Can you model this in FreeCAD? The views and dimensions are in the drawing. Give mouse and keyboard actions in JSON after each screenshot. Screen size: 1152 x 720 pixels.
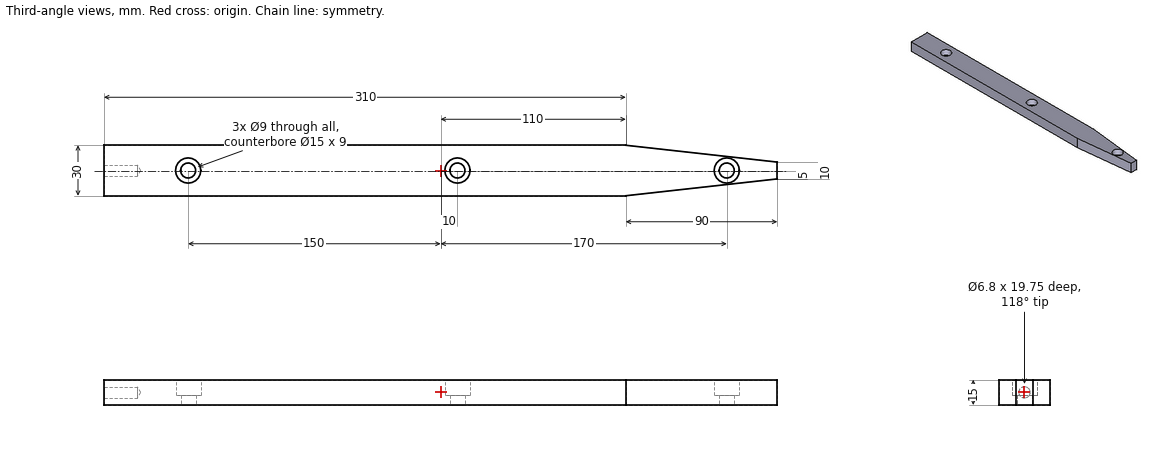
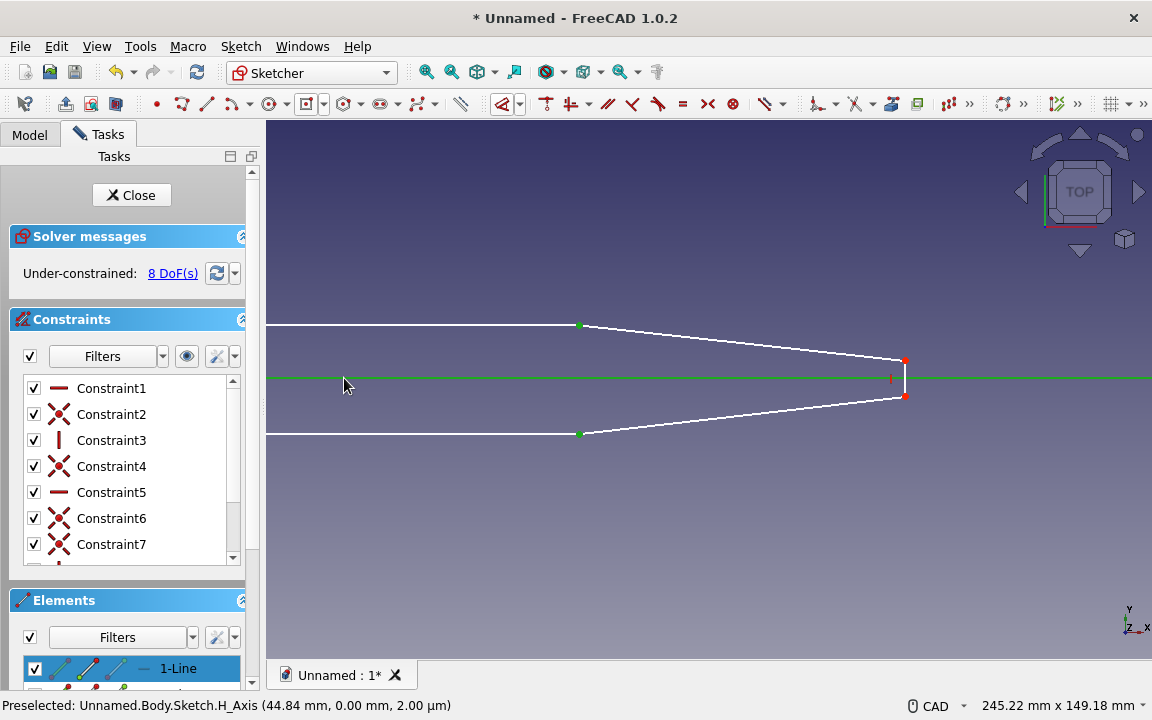
{"action": "key", "text": "s"}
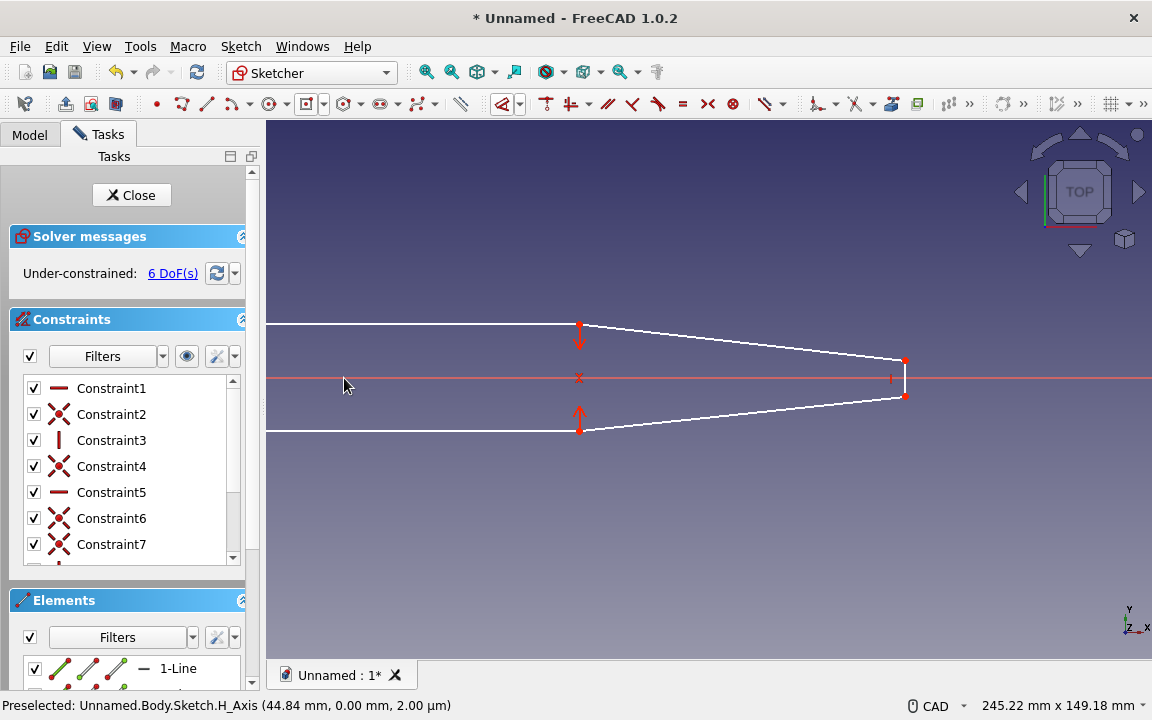
{"action": "left_click", "coordinate": [502, 104]}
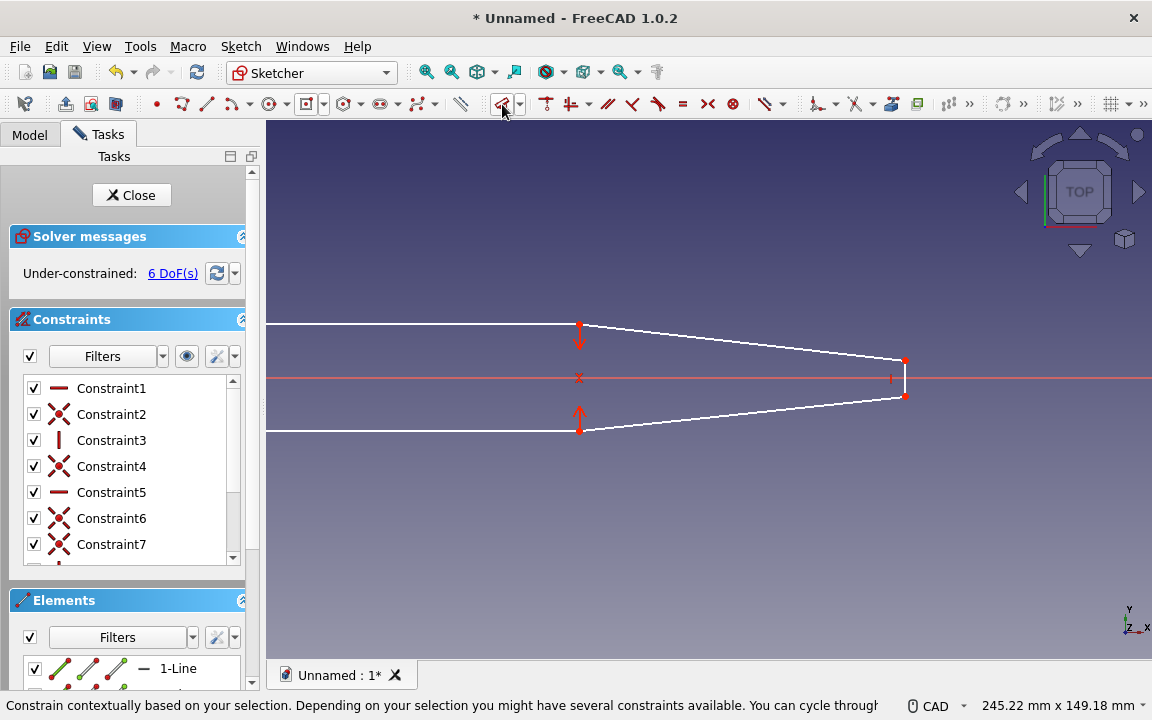
{"action": "scroll", "coordinate": [907, 396], "scroll_direction": "down", "scroll_amount": 5}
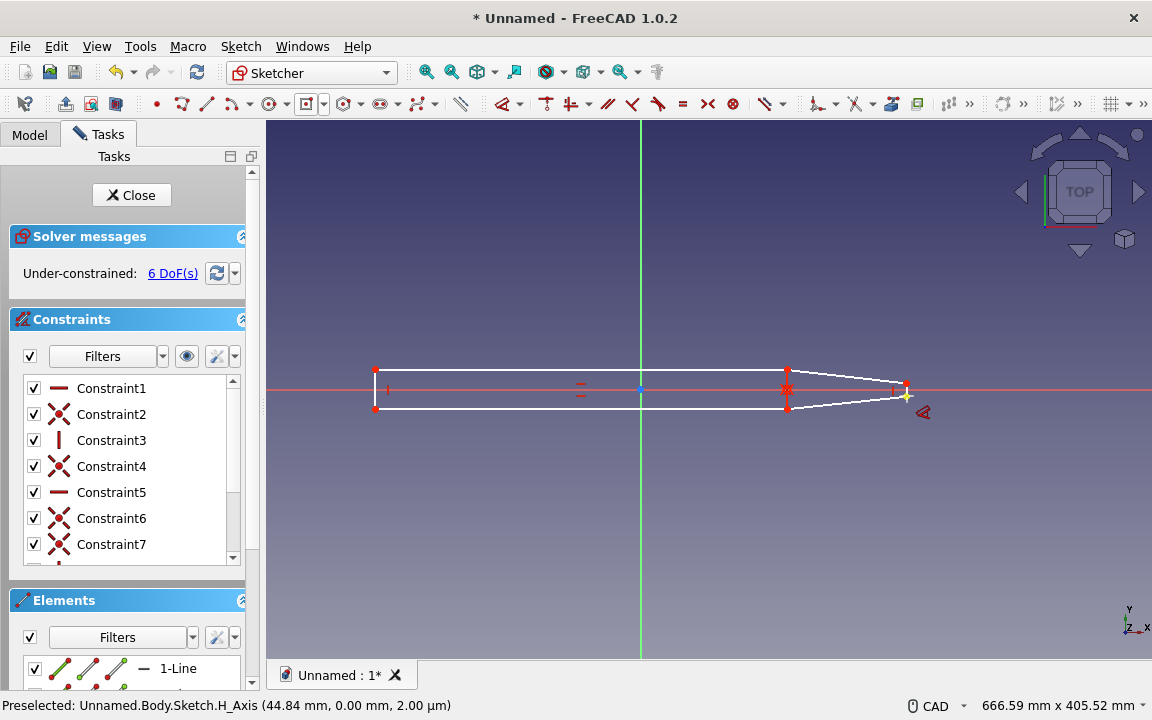
{"action": "scroll", "coordinate": [375, 382], "scroll_direction": "up", "scroll_amount": 3}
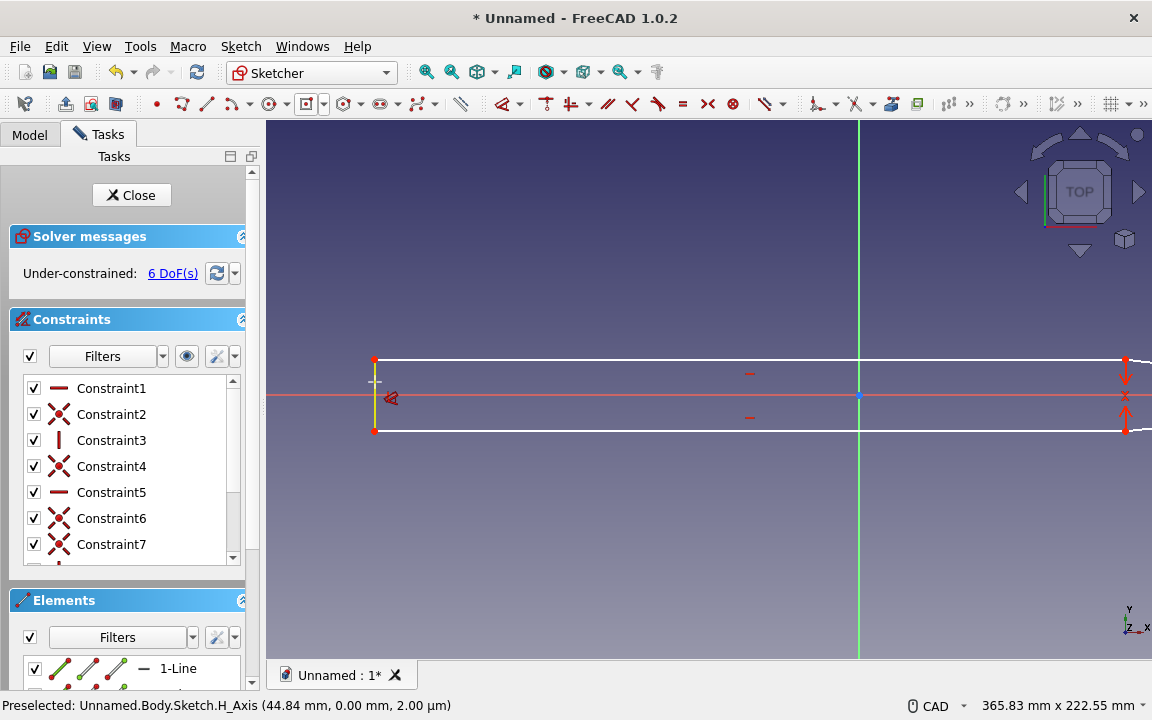
{"action": "left_click", "coordinate": [375, 381]}
{"action": "left_click", "coordinate": [341, 379]}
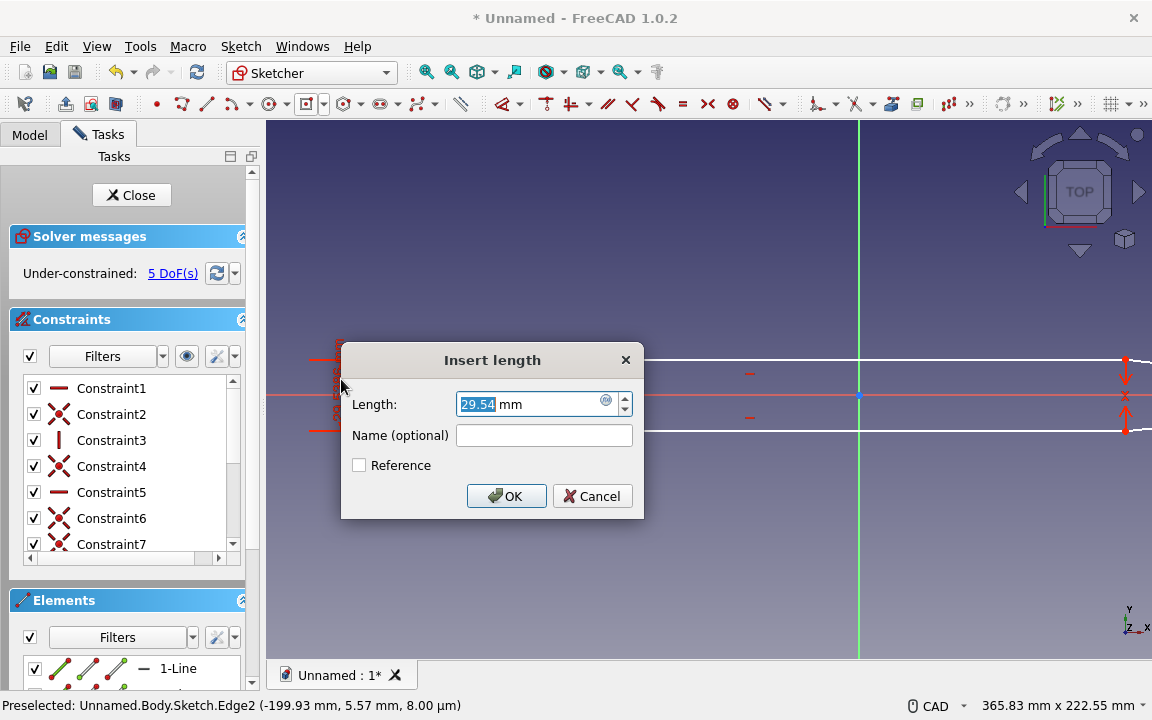
{"action": "type", "text": "30"}
{"action": "key", "text": "Return"}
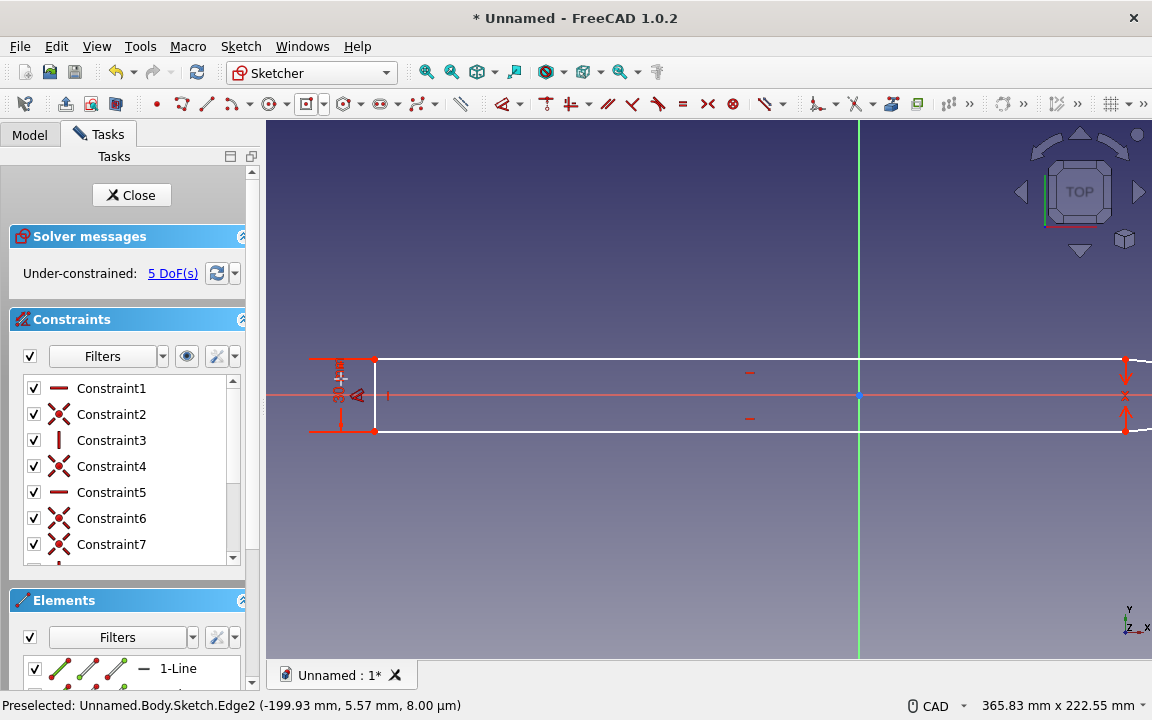
{"action": "scroll", "coordinate": [375, 382], "scroll_direction": "down", "scroll_amount": 3}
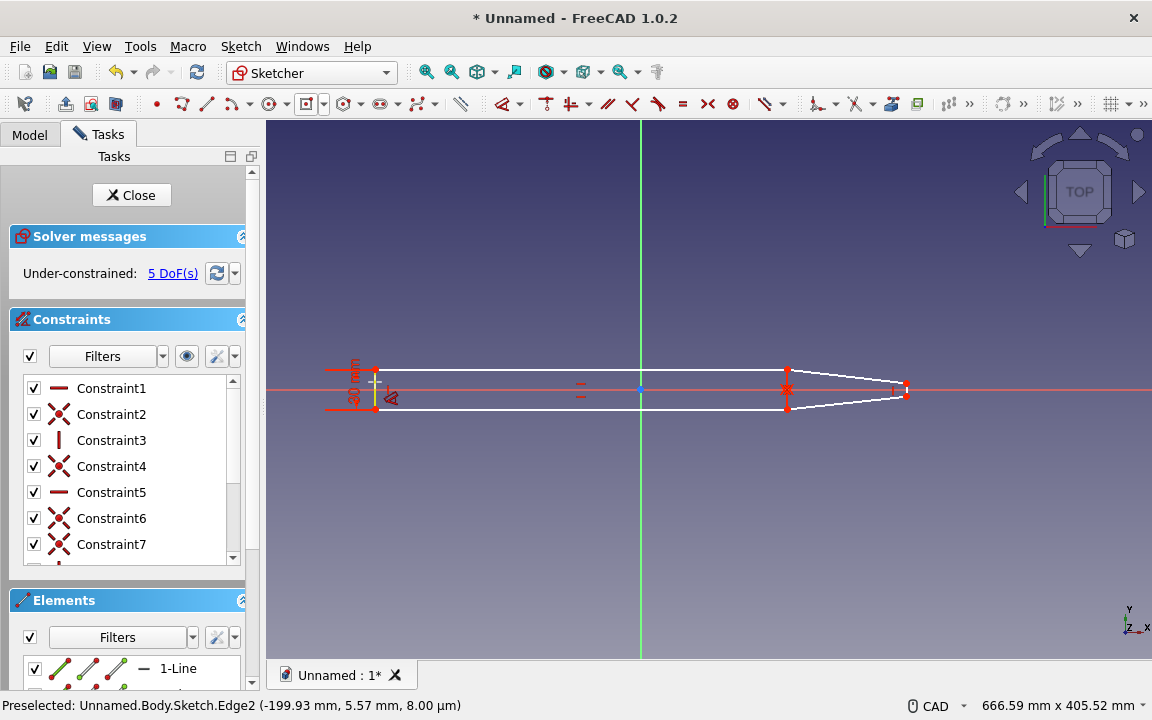
{"action": "scroll", "coordinate": [907, 391], "scroll_direction": "up", "scroll_amount": 6}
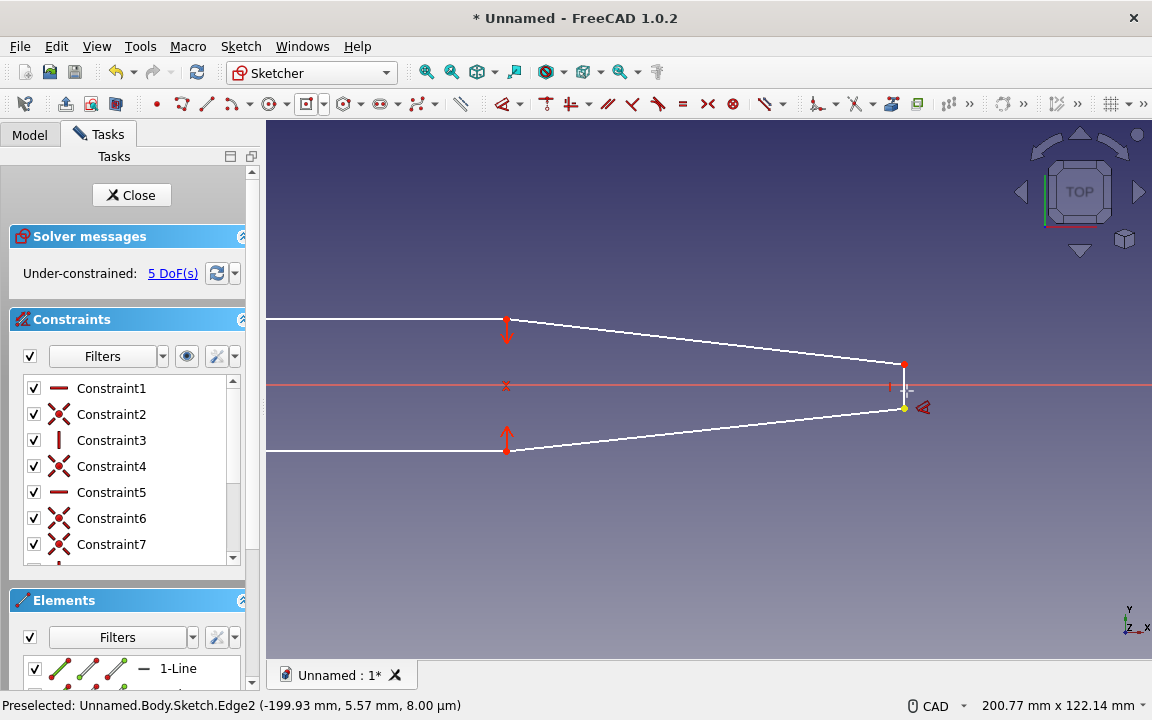
{"action": "left_click", "coordinate": [904, 391]}
{"action": "left_click", "coordinate": [938, 371]}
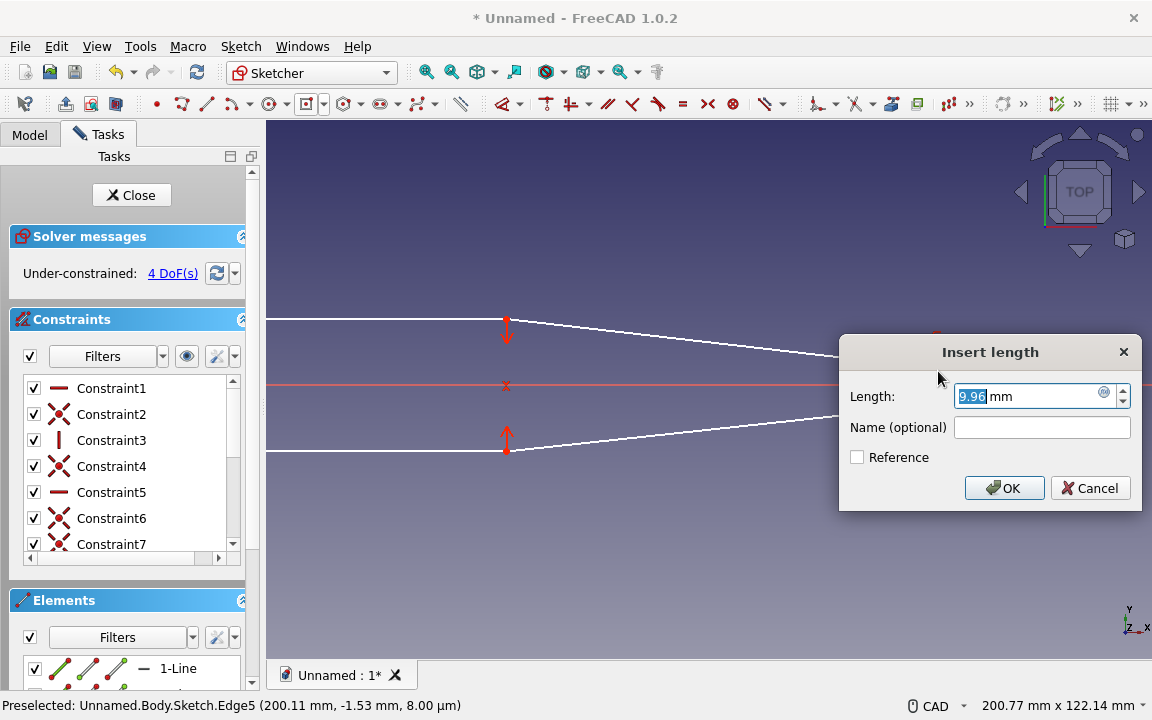
{"action": "type", "text": "10"}
{"action": "key", "text": "Return"}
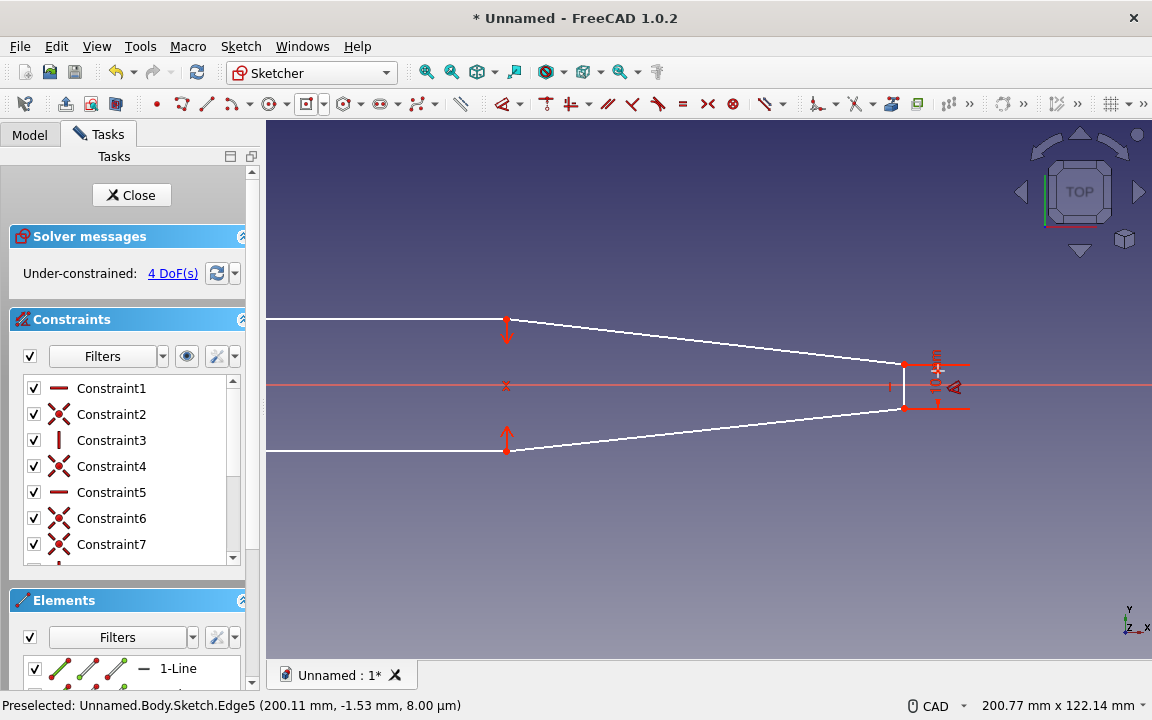
{"action": "scroll", "coordinate": [904, 409], "scroll_direction": "up", "scroll_amount": 3}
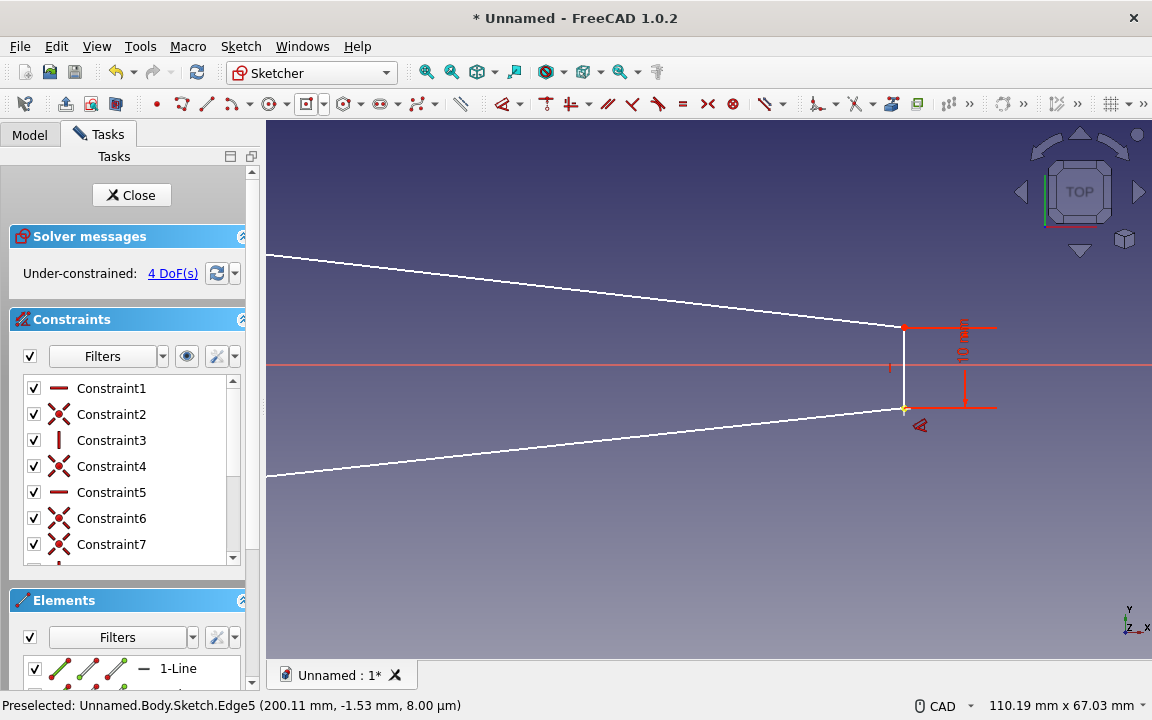
{"action": "left_click", "coordinate": [904, 408]}
{"action": "left_click", "coordinate": [938, 387]}